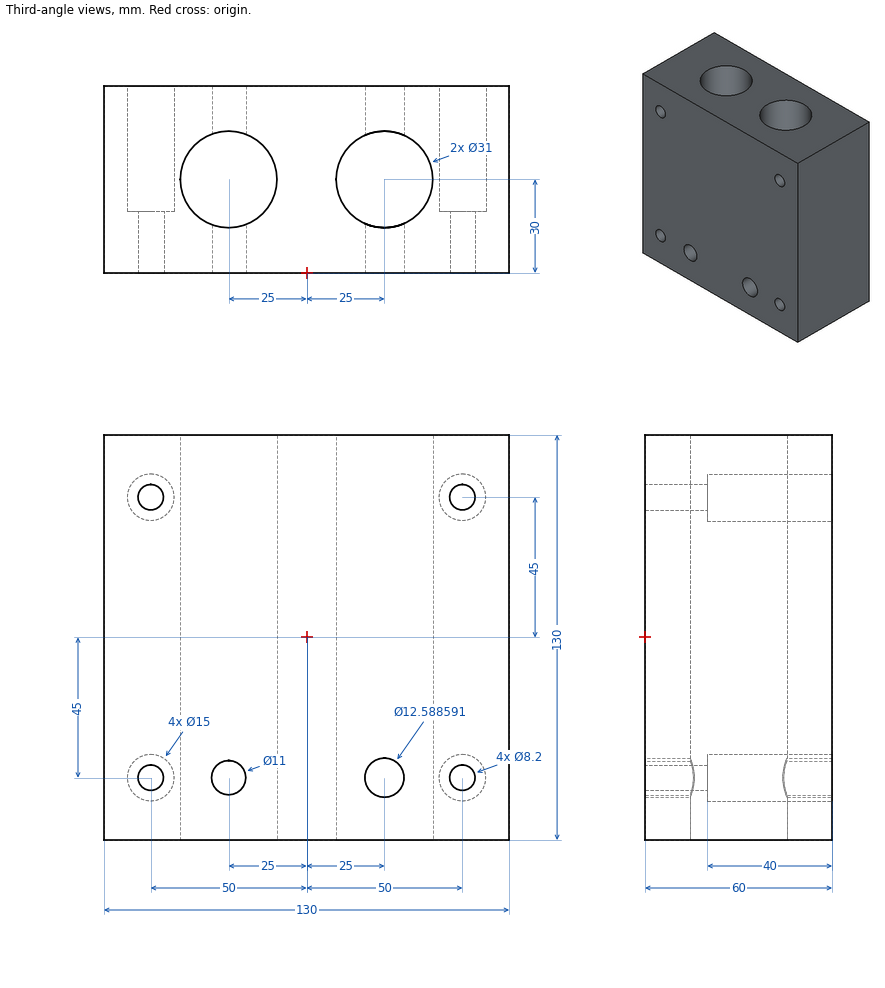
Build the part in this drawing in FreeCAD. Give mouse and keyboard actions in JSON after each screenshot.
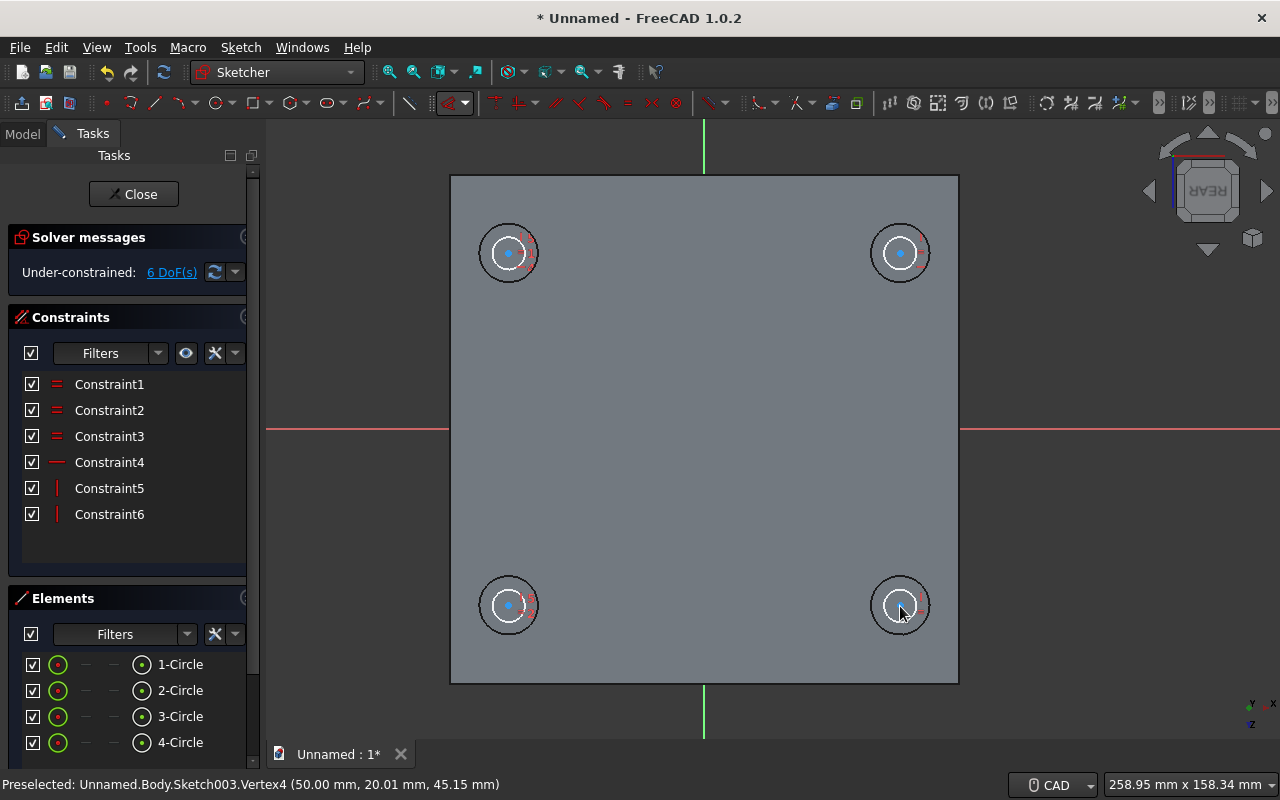
{"action": "left_click", "coordinate": [509, 606]}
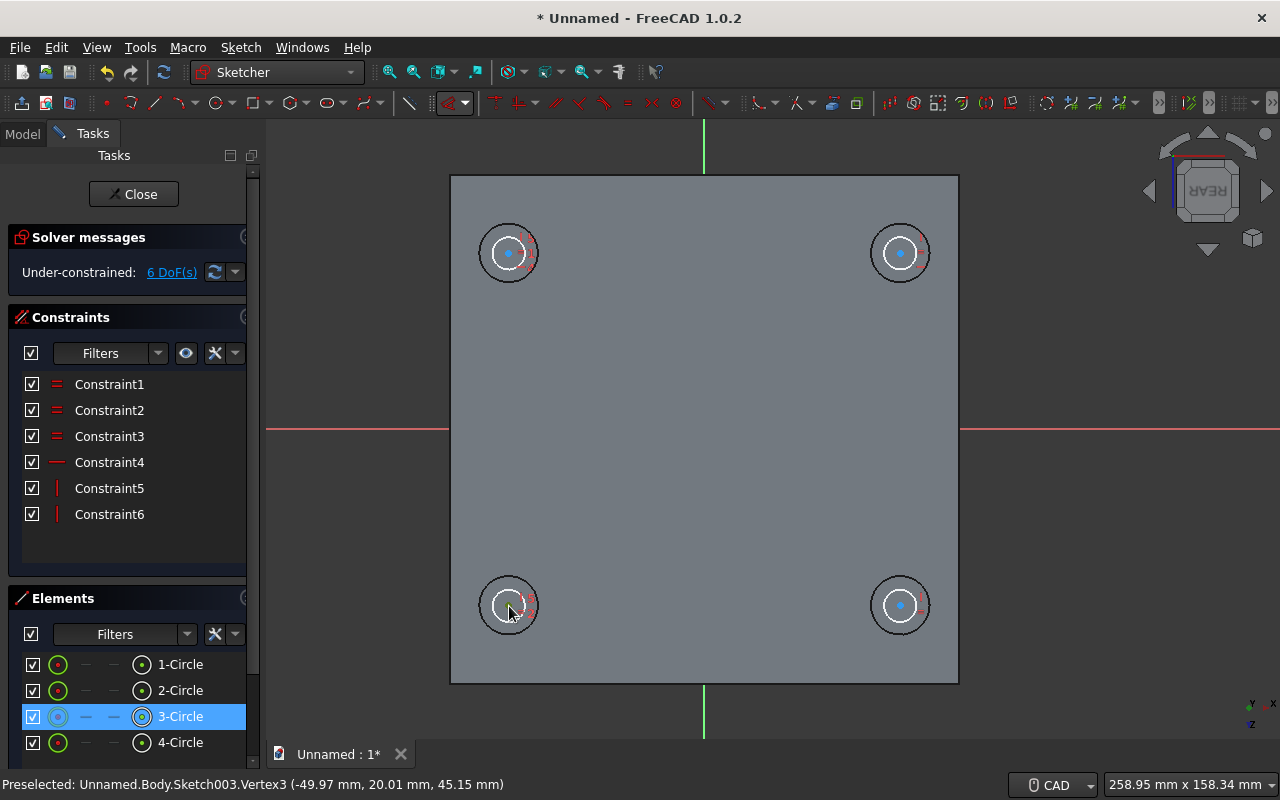
{"action": "left_click", "coordinate": [900, 606]}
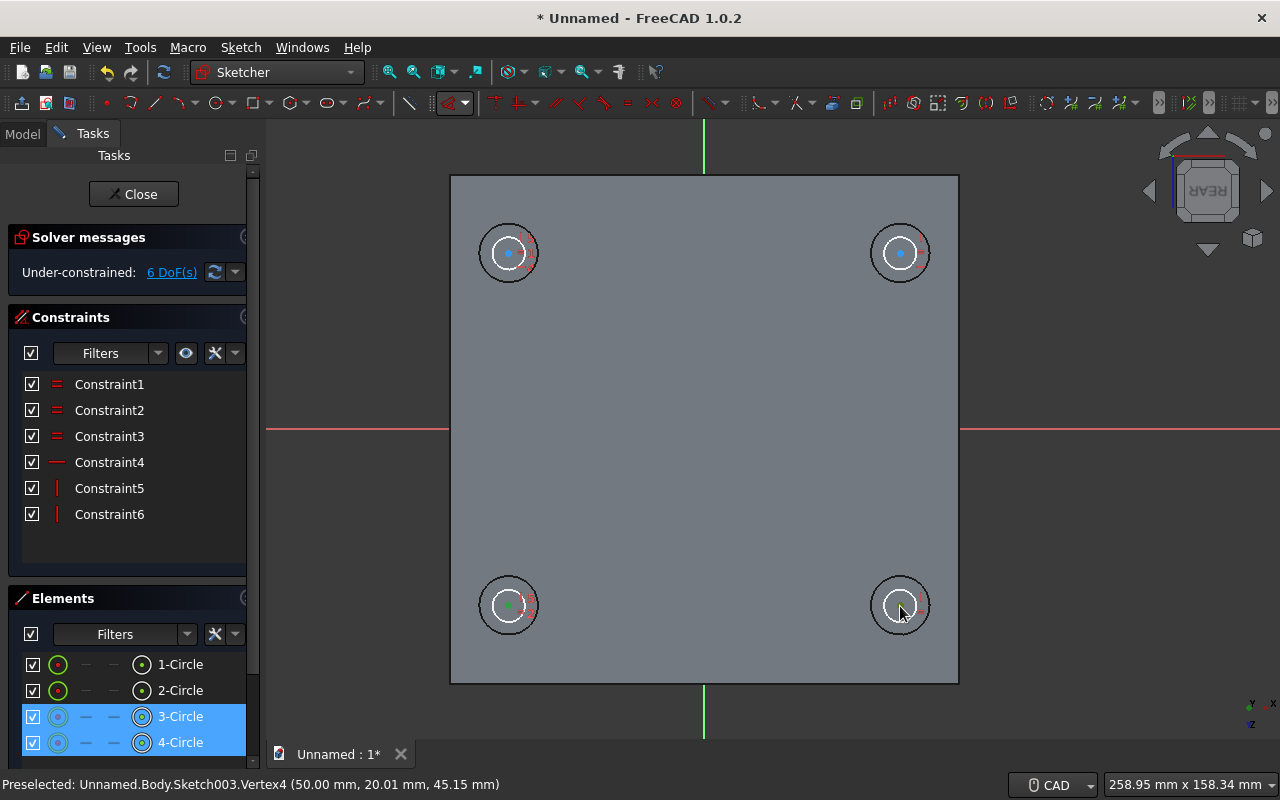
{"action": "key", "text": "h"}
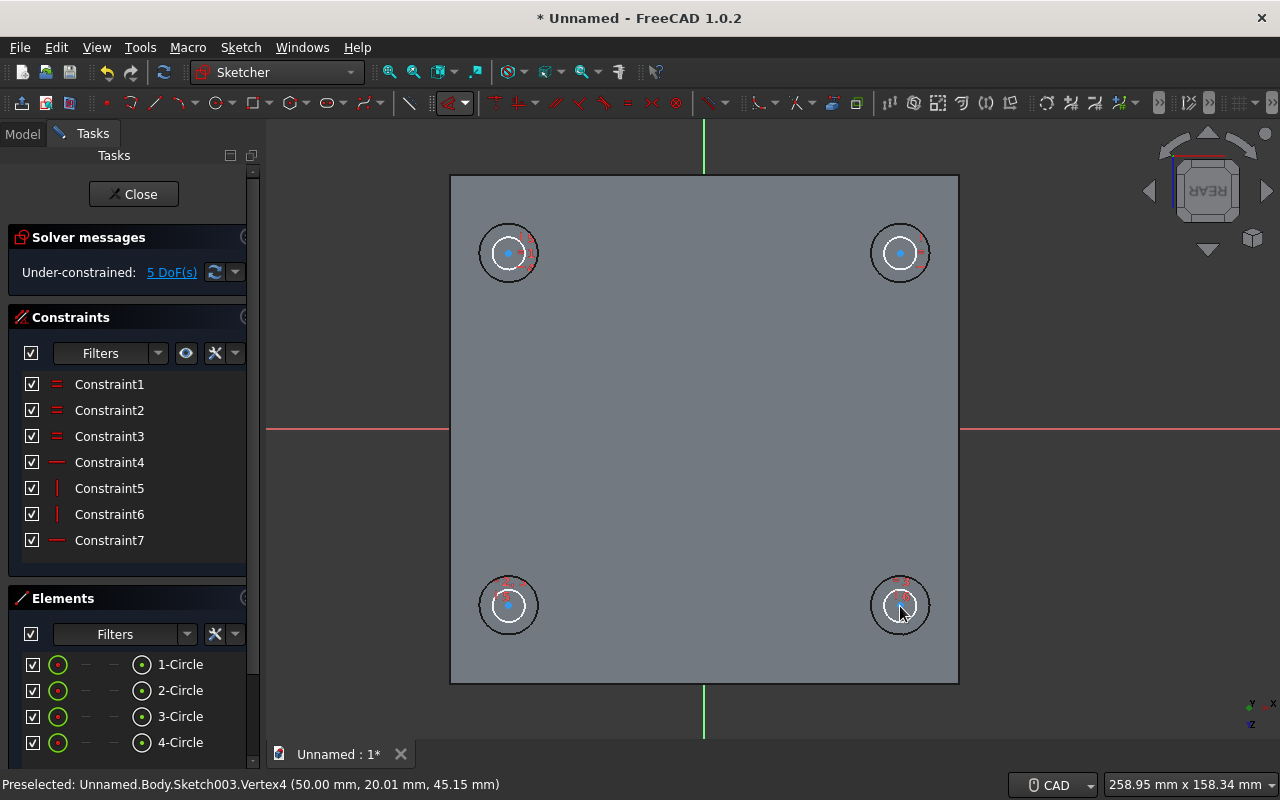
{"action": "scroll", "coordinate": [912, 242], "scroll_direction": "up", "scroll_amount": 2}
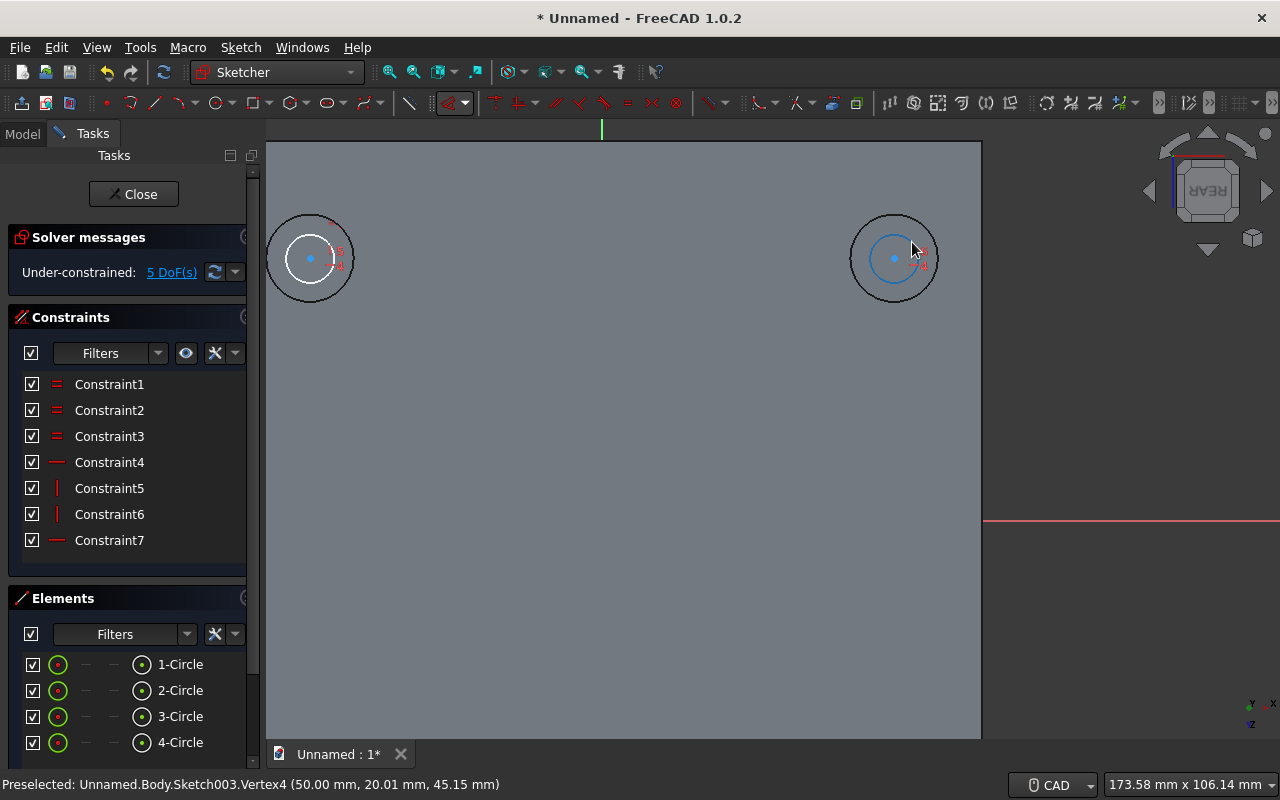
{"action": "left_click", "coordinate": [911, 242]}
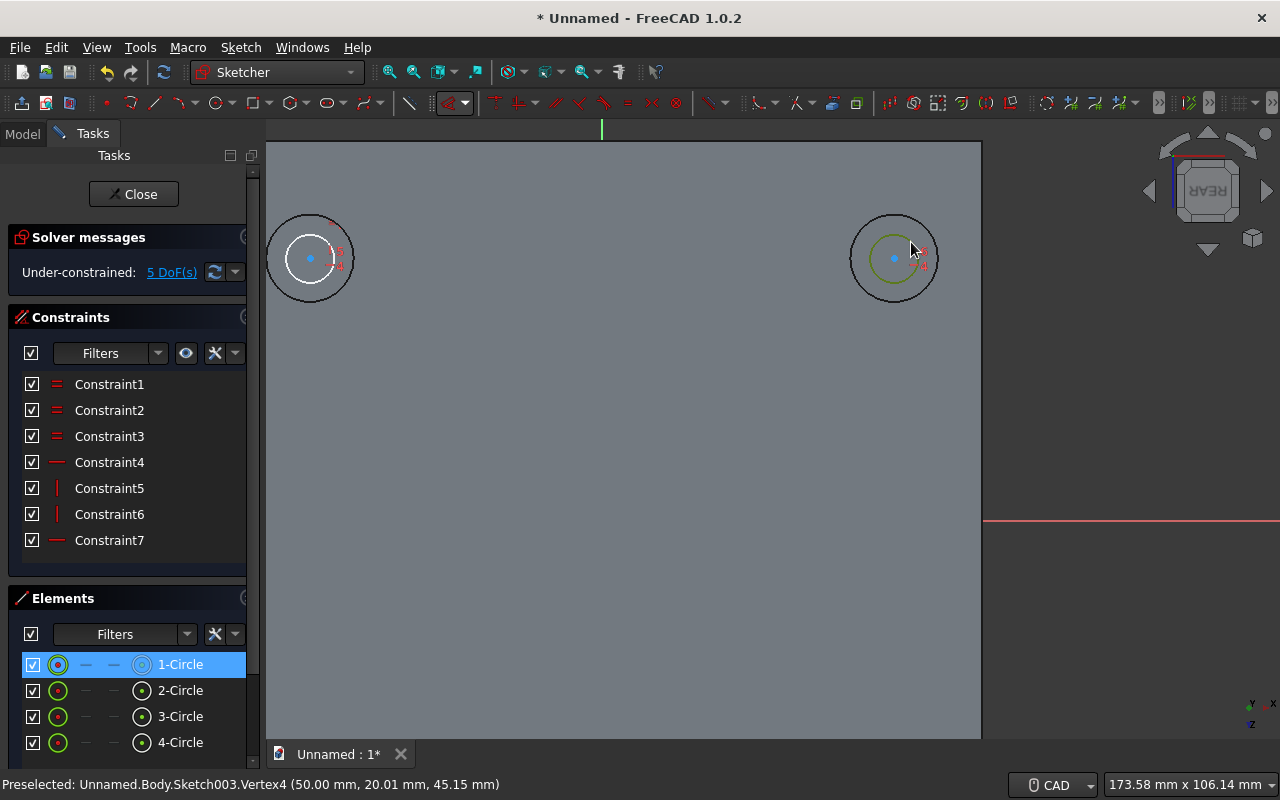
{"action": "key", "text": "k o"}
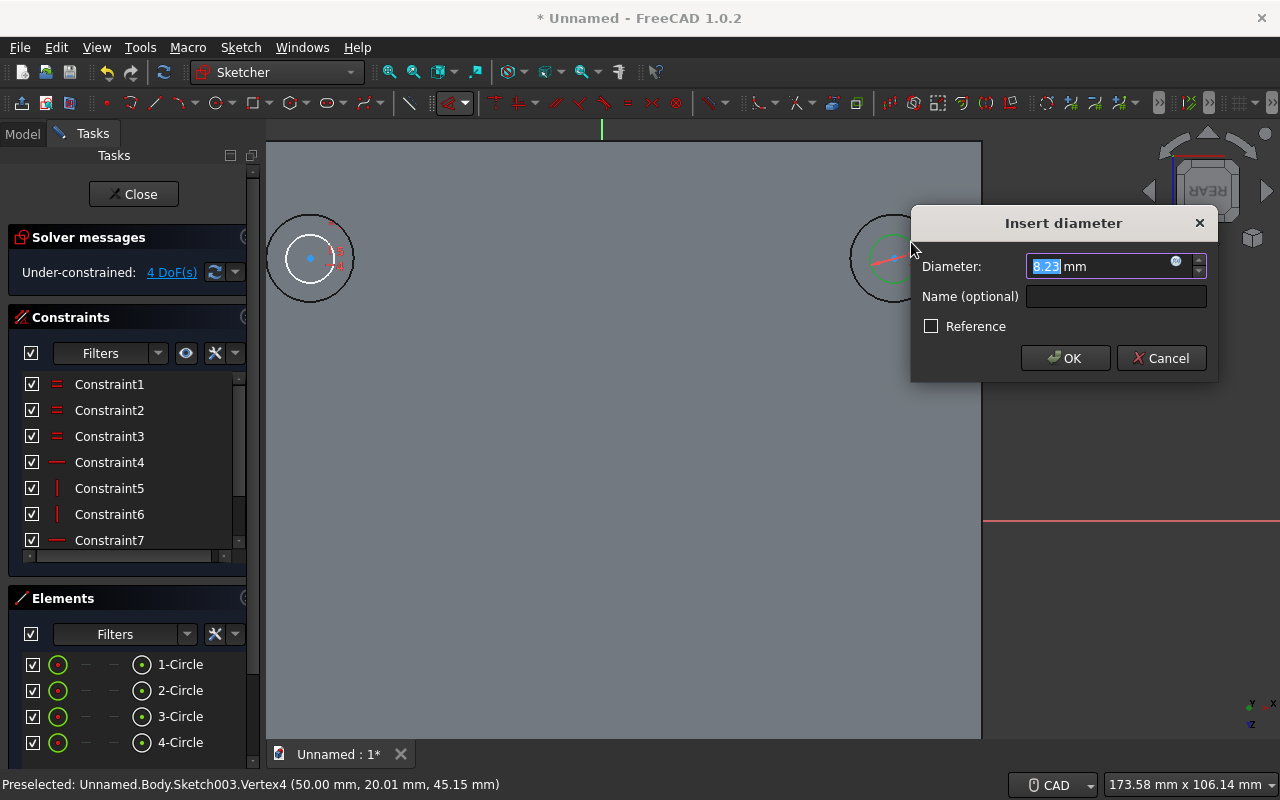
{"action": "type", "text": "8.2"}
{"action": "key", "text": "Return"}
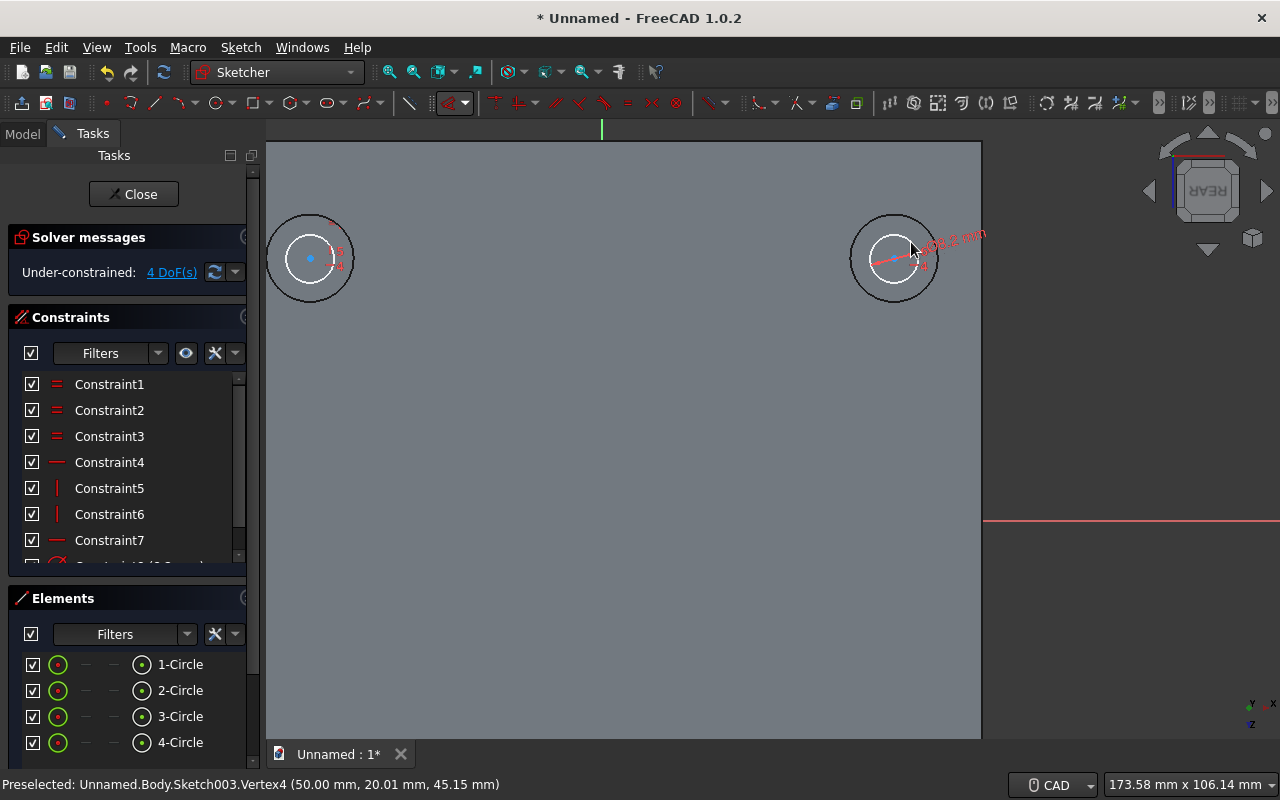
{"action": "left_click", "coordinate": [894, 259]}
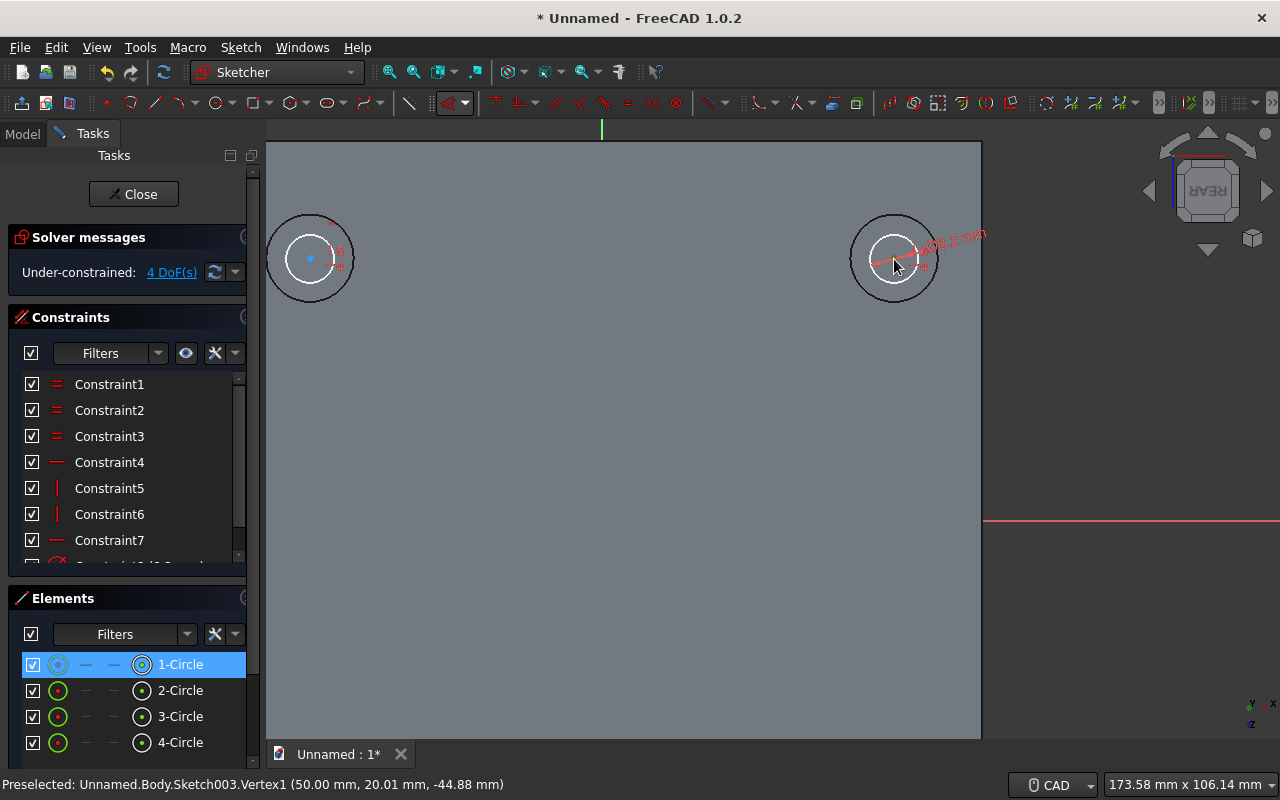
{"action": "key", "text": "l"}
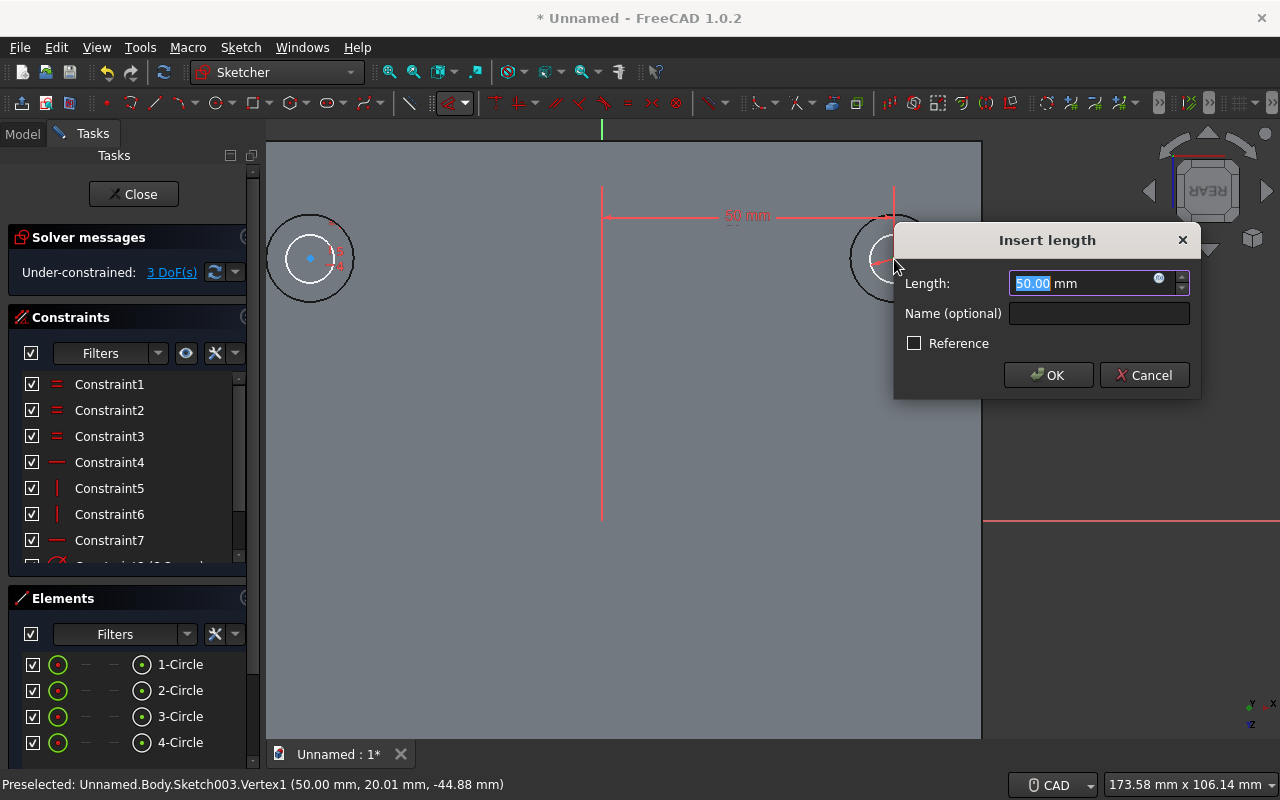
{"action": "type", "text": "50"}
{"action": "key", "text": "Return"}